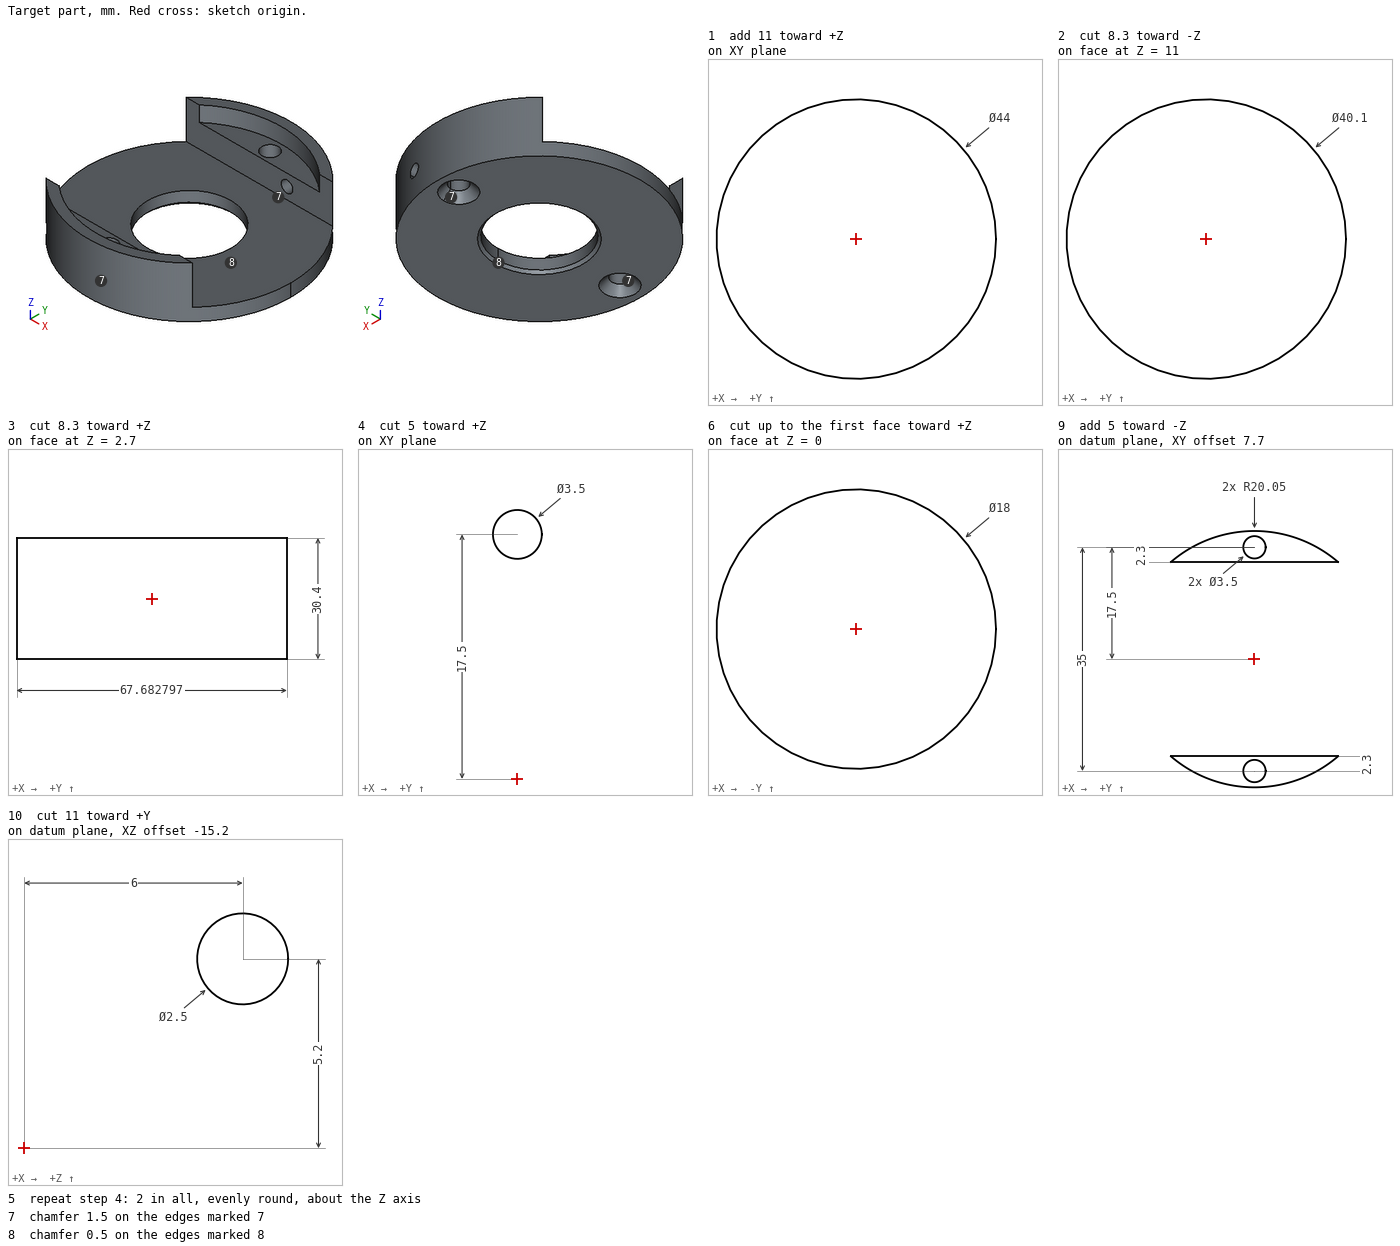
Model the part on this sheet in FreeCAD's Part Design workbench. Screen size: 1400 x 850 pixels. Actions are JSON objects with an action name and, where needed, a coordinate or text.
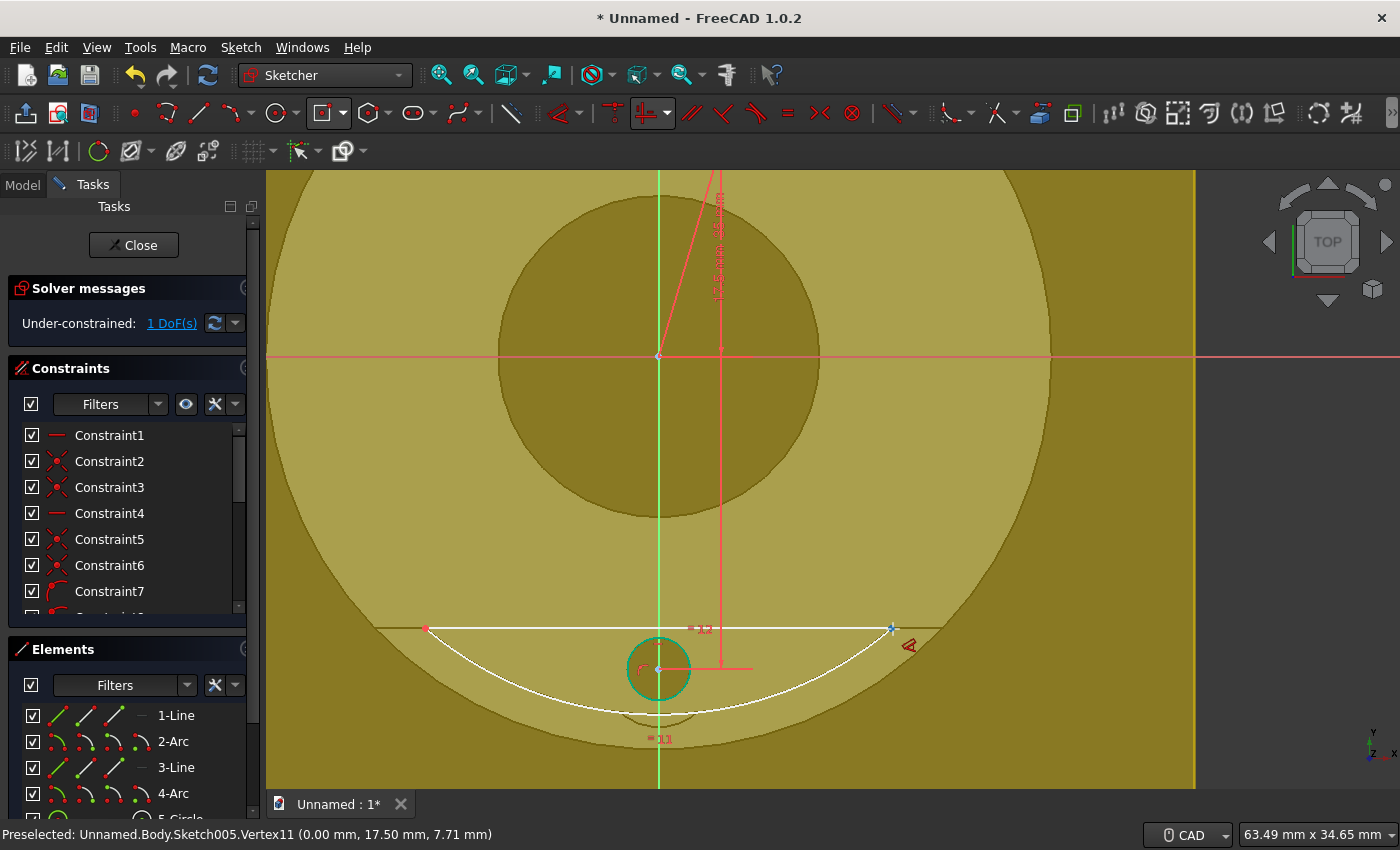
{"action": "left_click", "coordinate": [892, 628]}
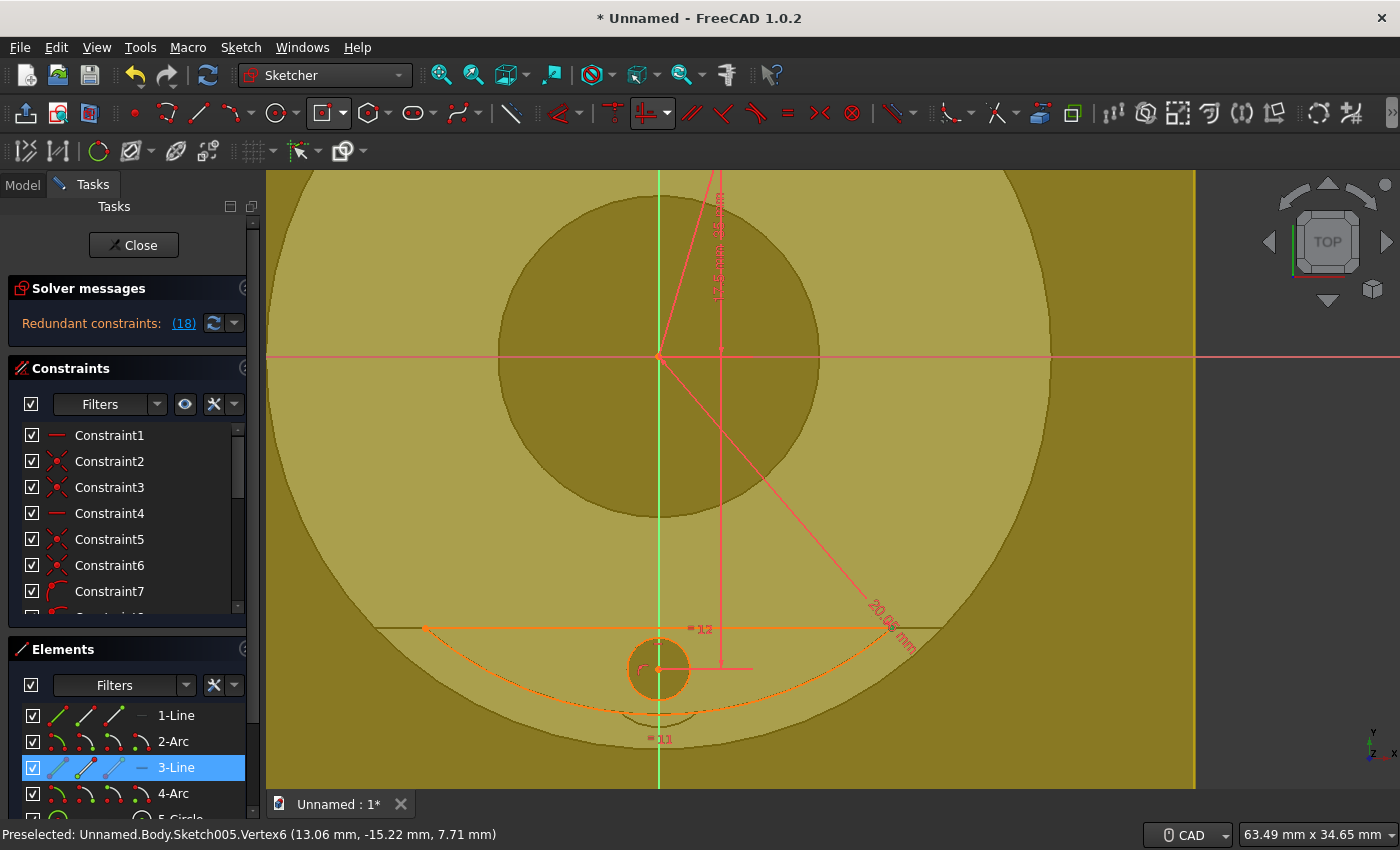
{"action": "left_click", "coordinate": [659, 669]}
{"action": "left_click", "coordinate": [926, 649]}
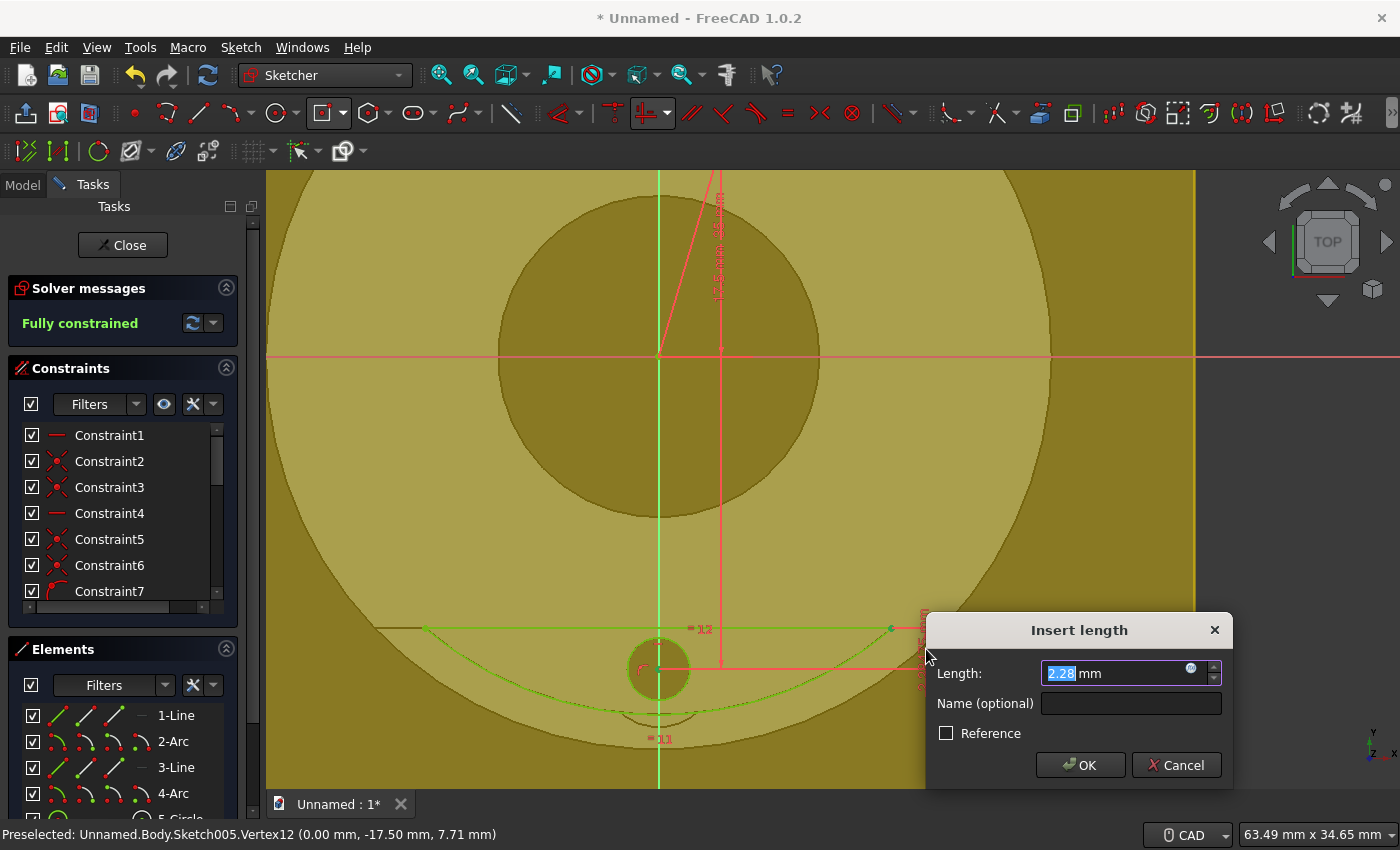
{"action": "type", "text": "2.3"}
{"action": "key", "text": "Return"}
{"action": "key", "text": "Escape"}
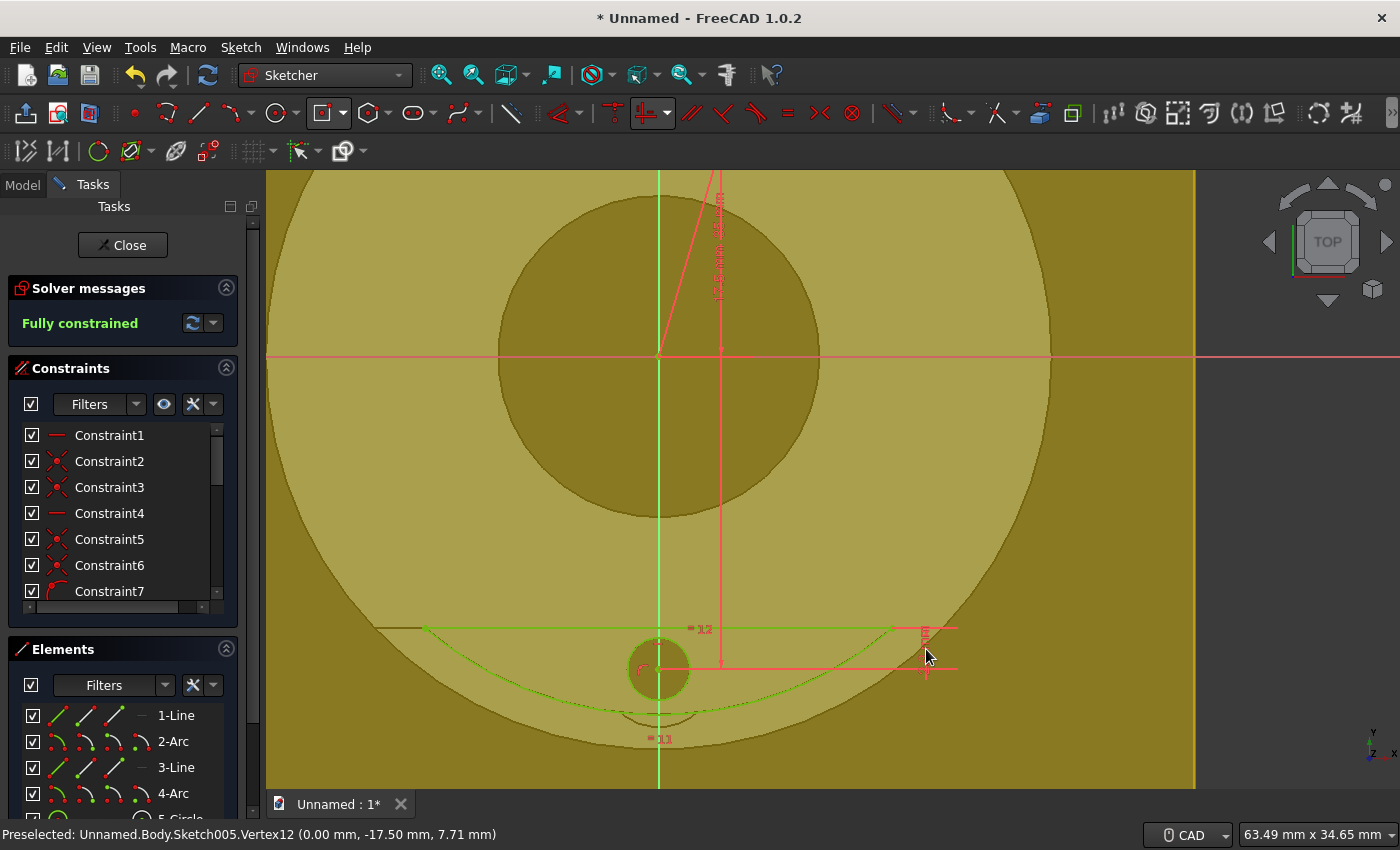
{"action": "left_click", "coordinate": [123, 245]}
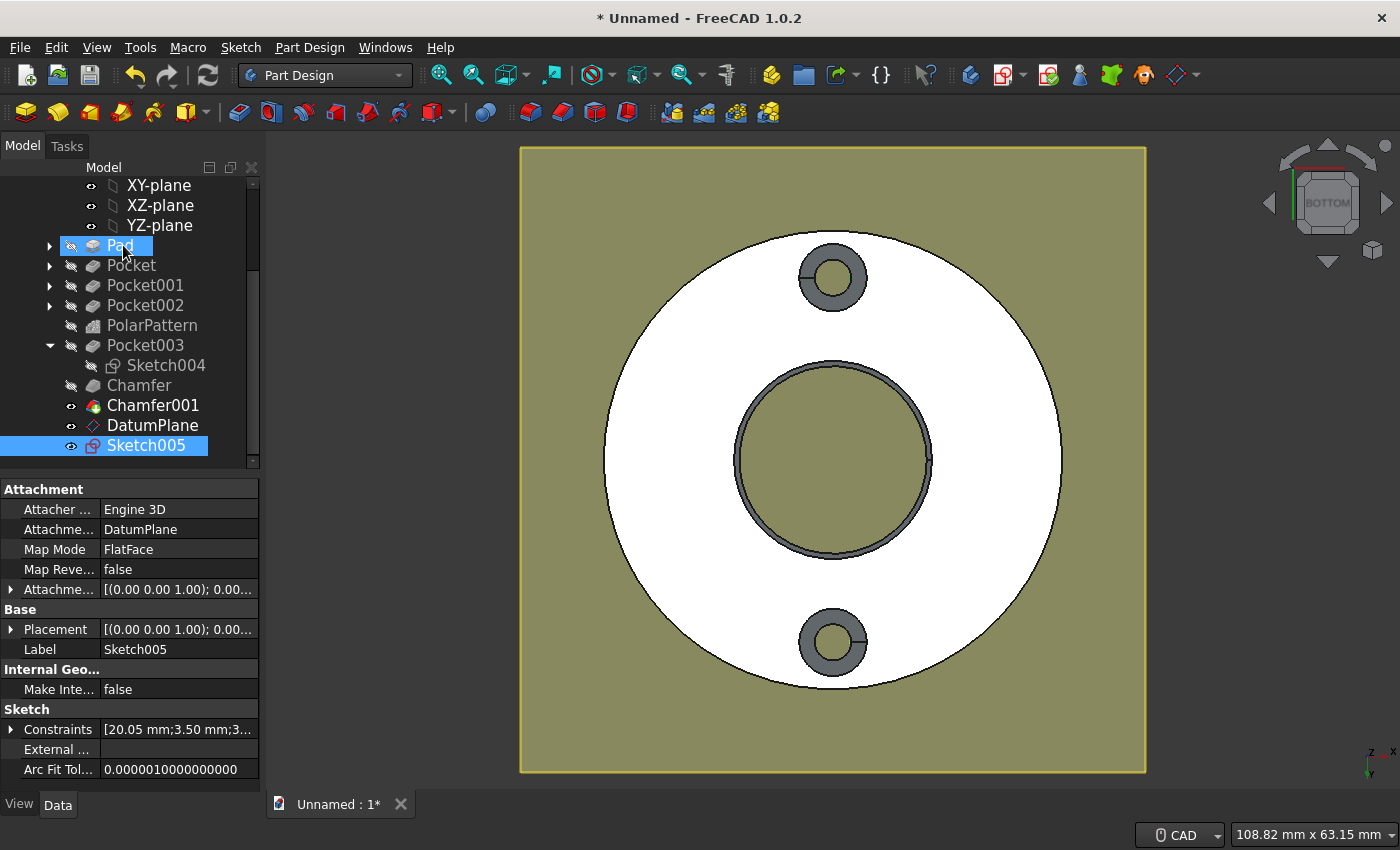
{"action": "left_click", "coordinate": [26, 112]}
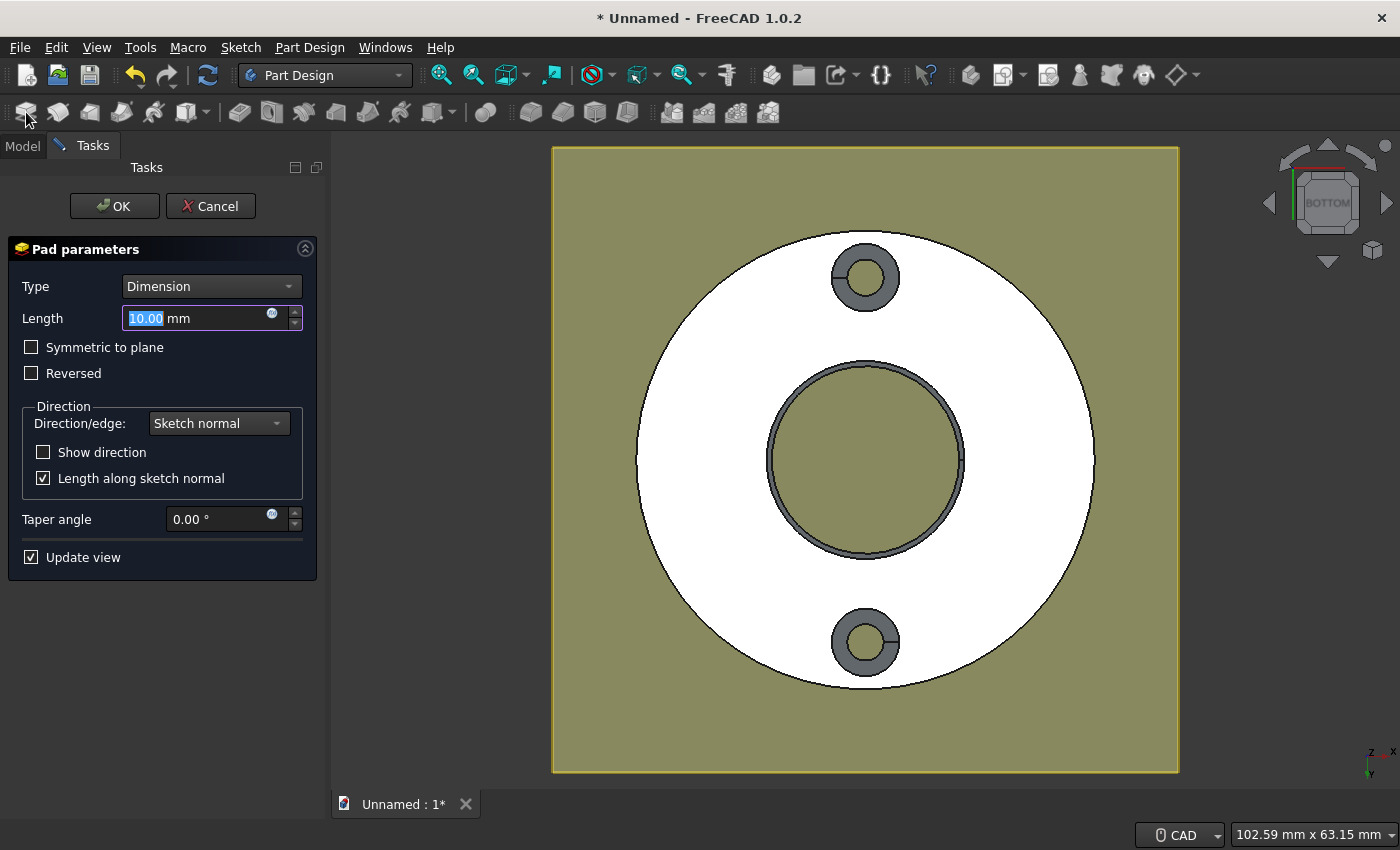
{"action": "type", "text": "5"}
{"action": "key", "text": "Tab"}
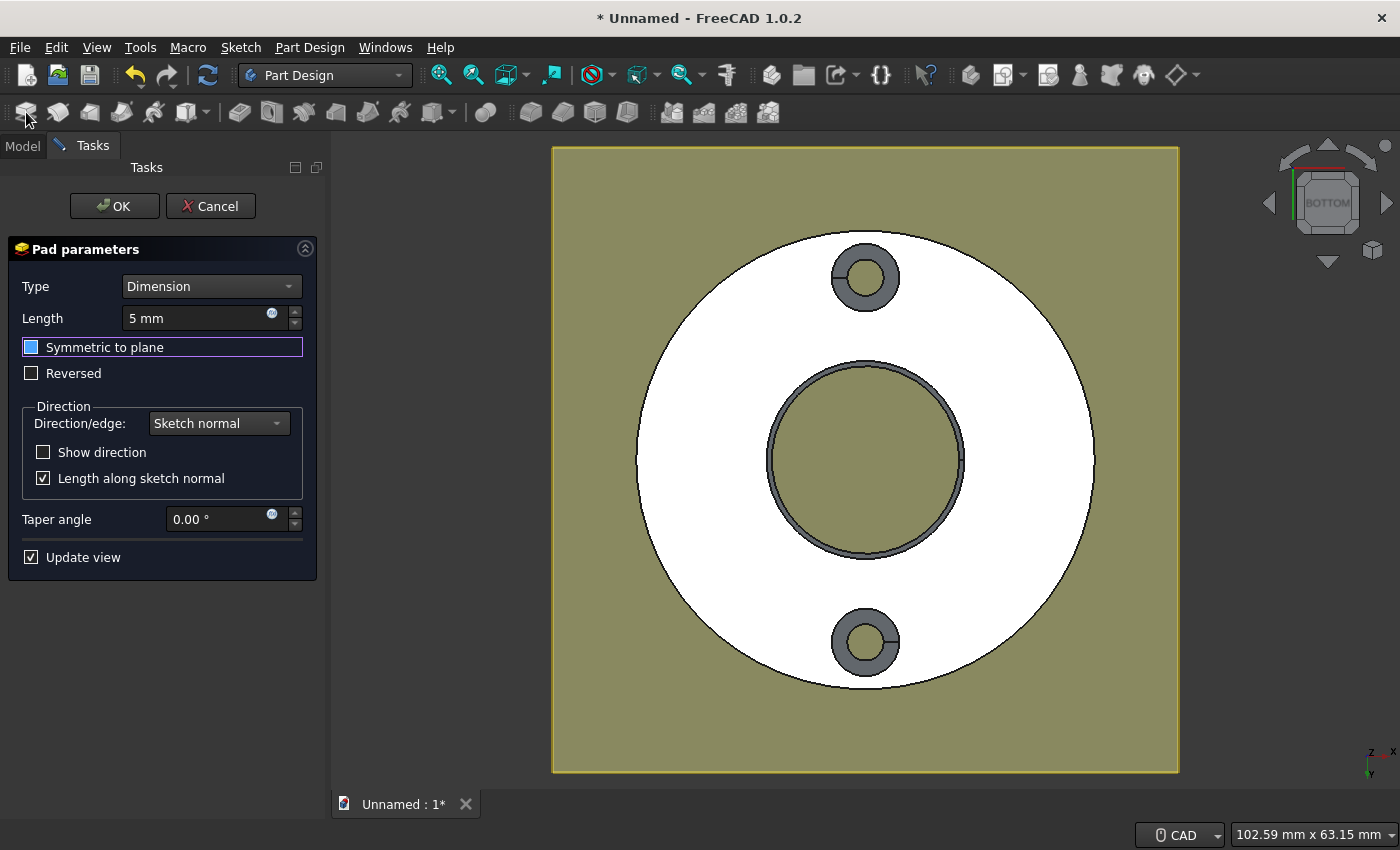
{"action": "left_click", "coordinate": [30, 373]}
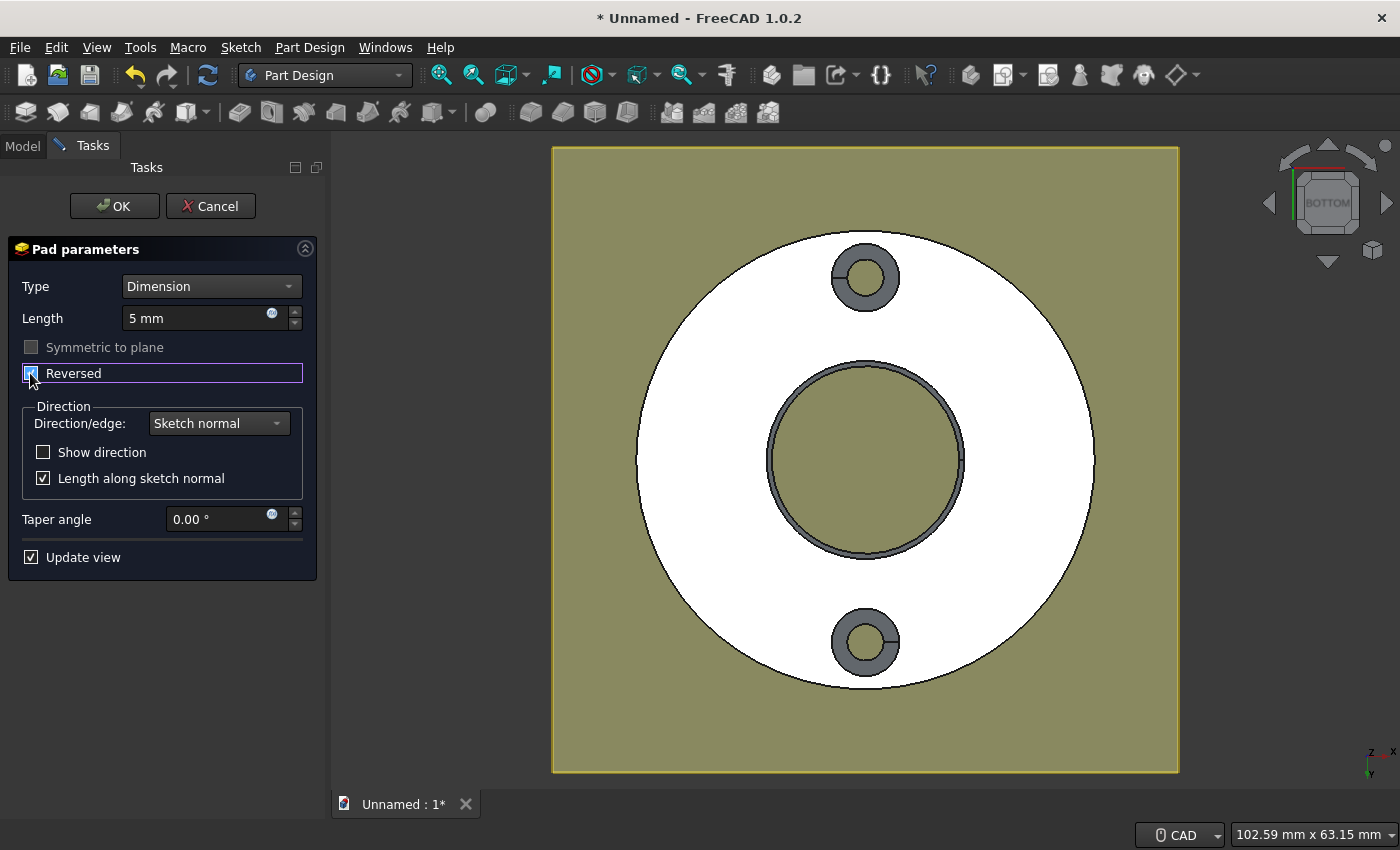
{"action": "left_click", "coordinate": [115, 206]}